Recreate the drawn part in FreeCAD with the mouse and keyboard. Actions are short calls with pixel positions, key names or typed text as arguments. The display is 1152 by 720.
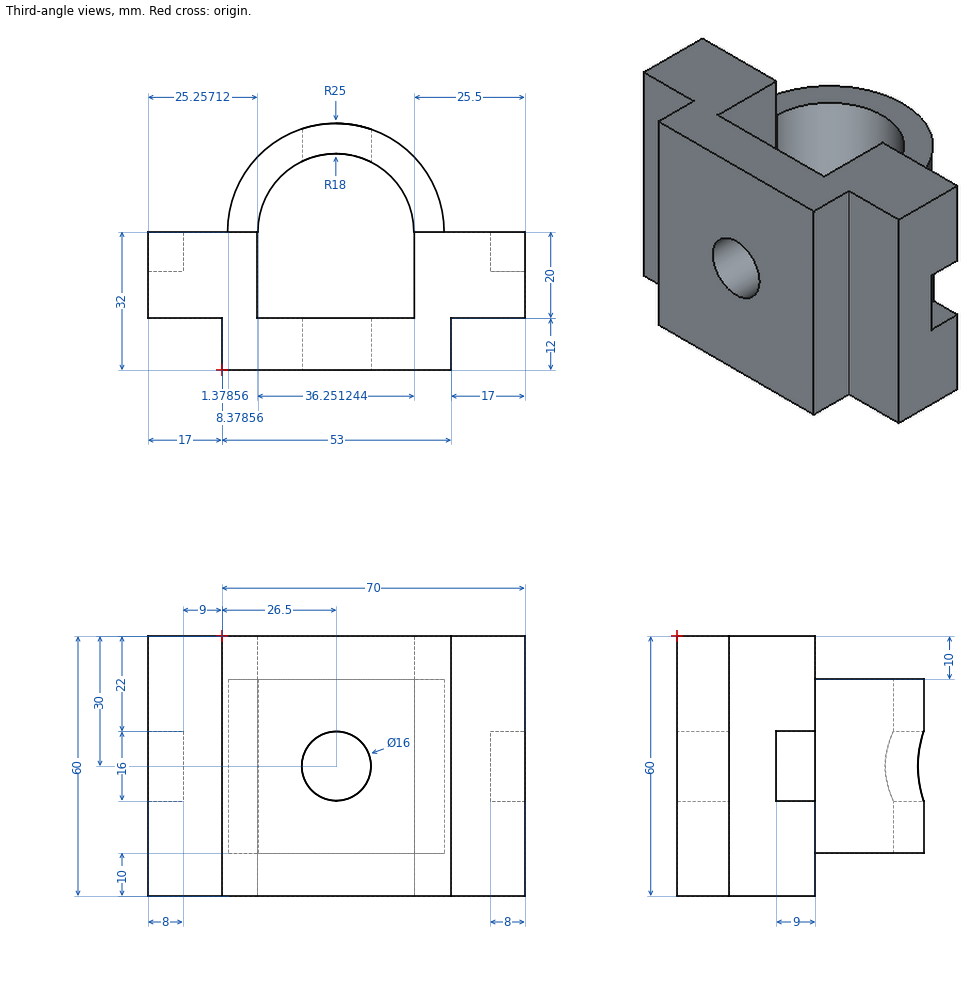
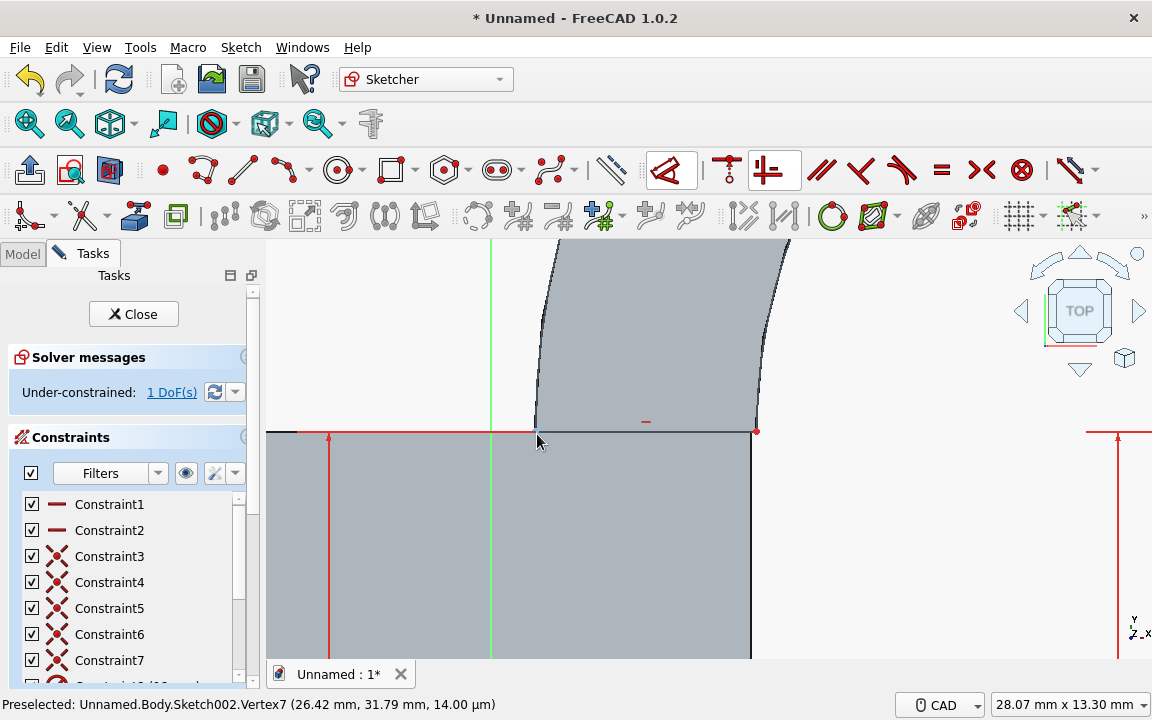
click(536, 432)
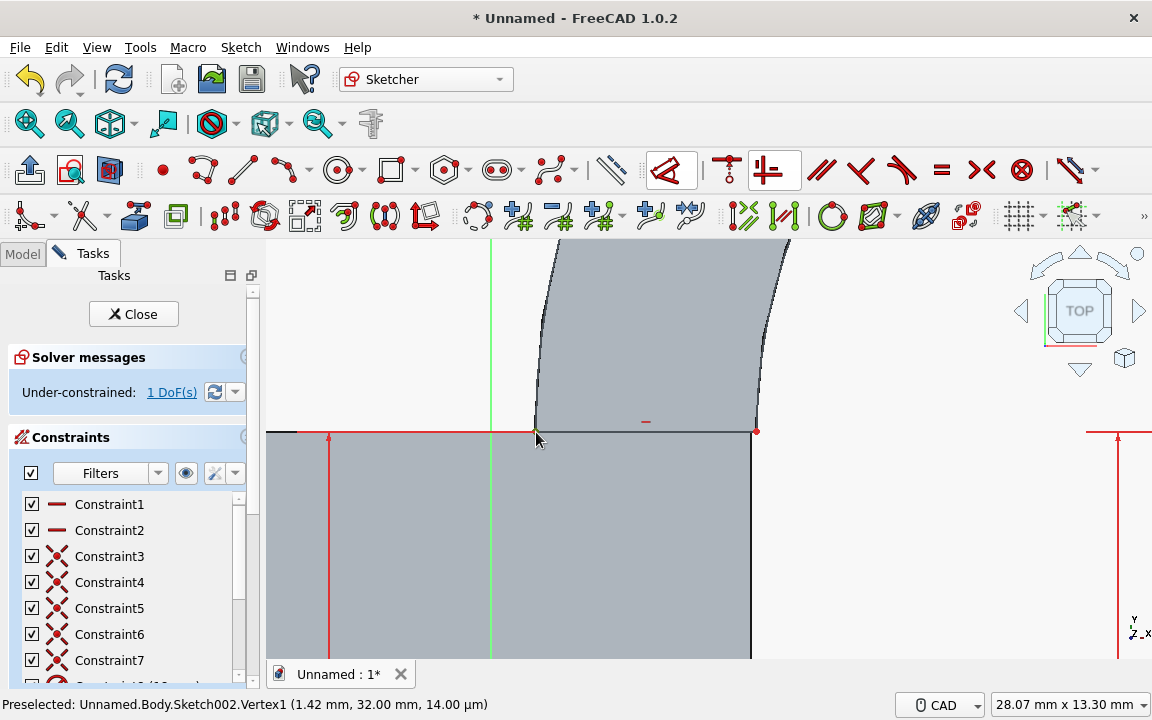
key(l)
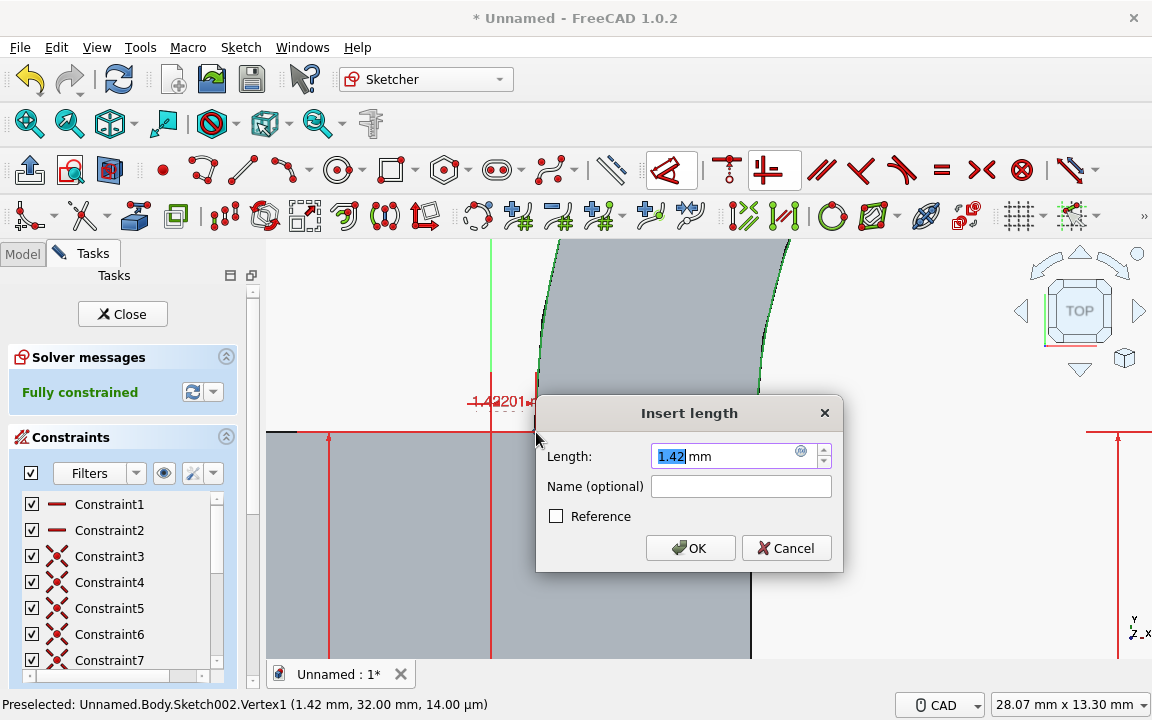
text(1.37856)
key(Return)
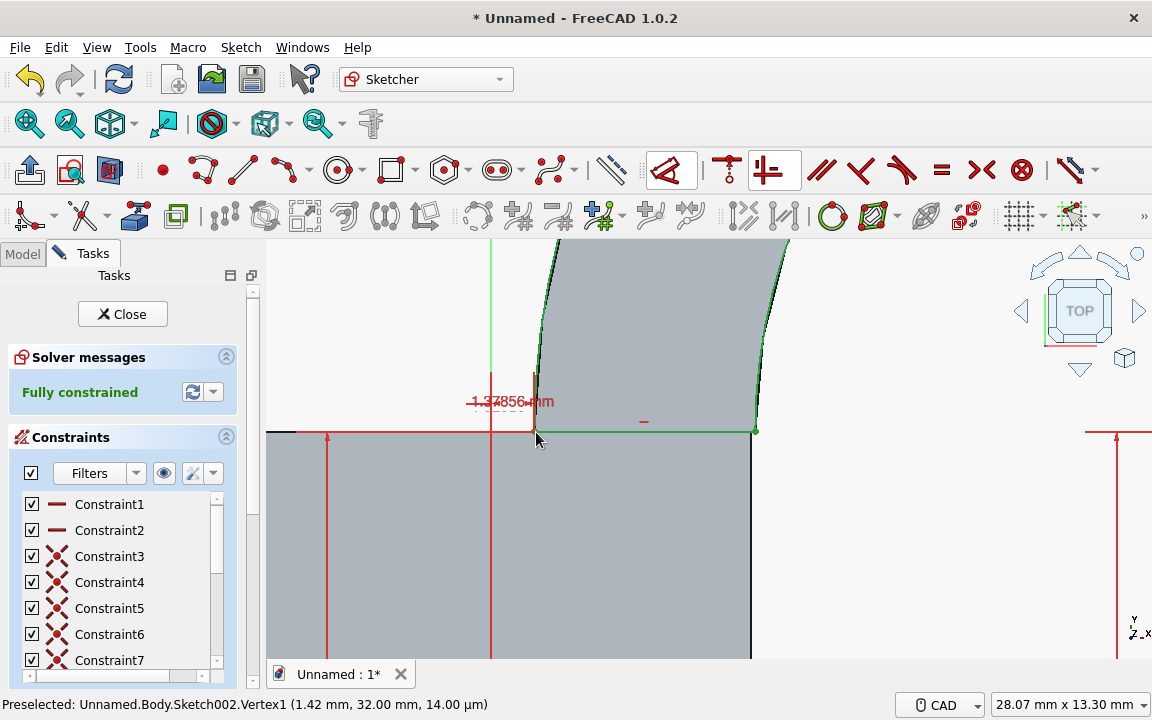
click(123, 314)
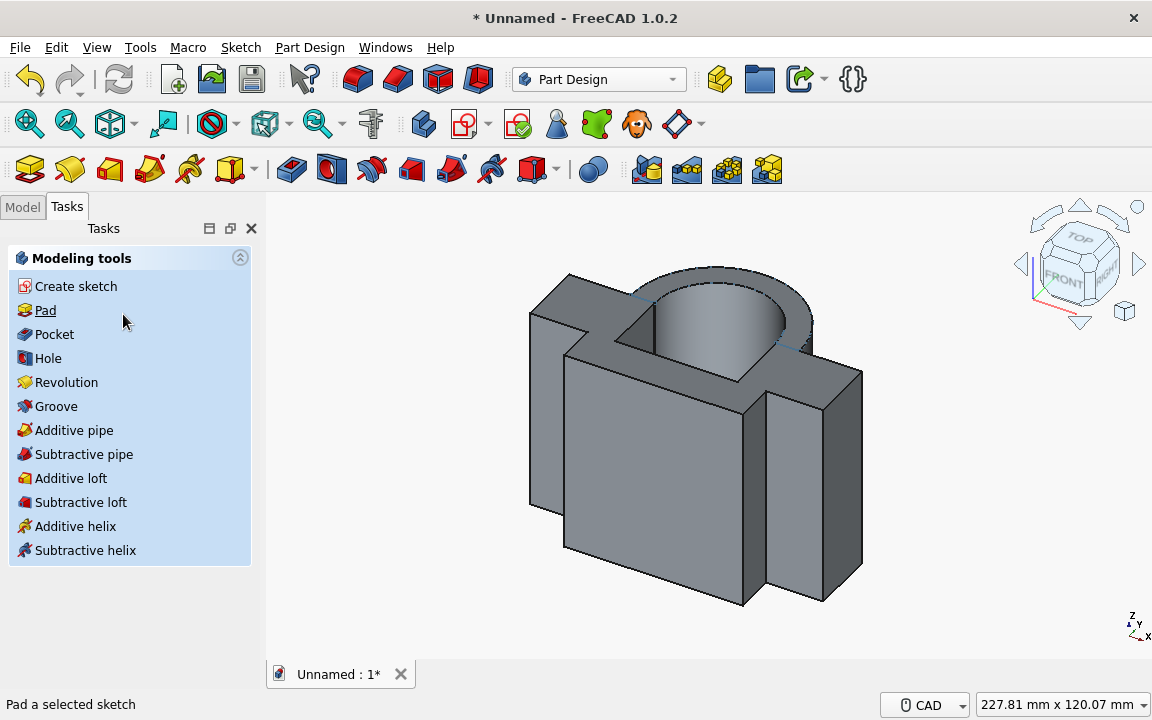
click(292, 170)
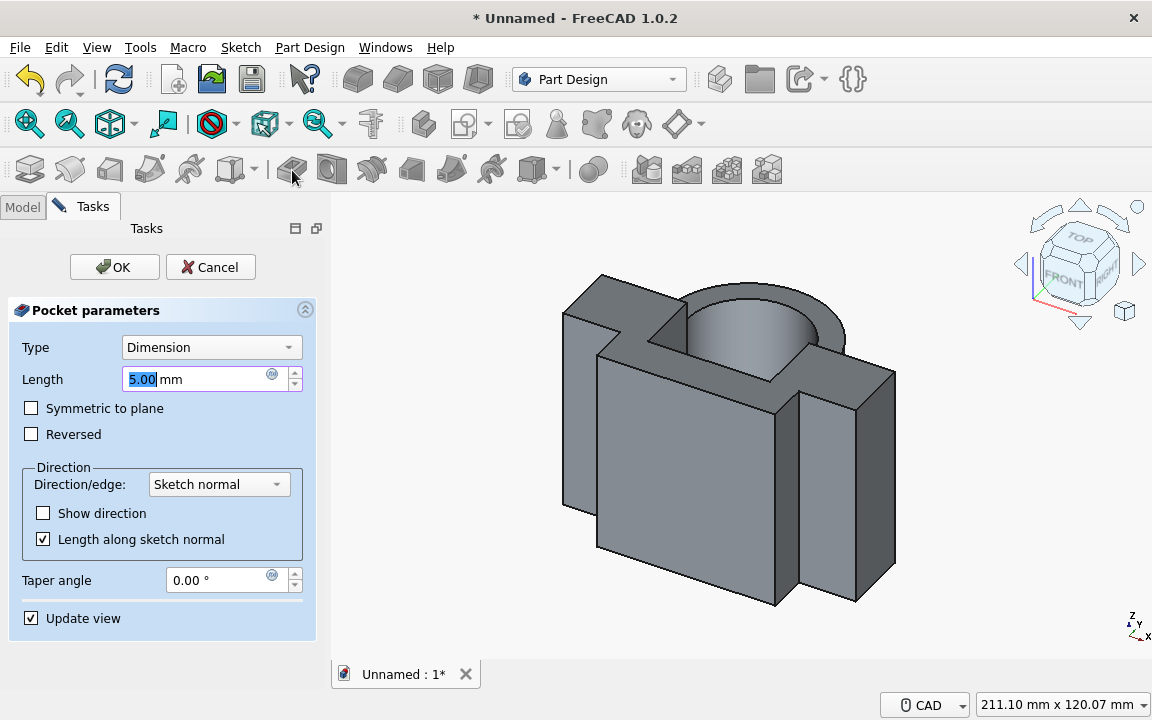
text(10)
key(Tab)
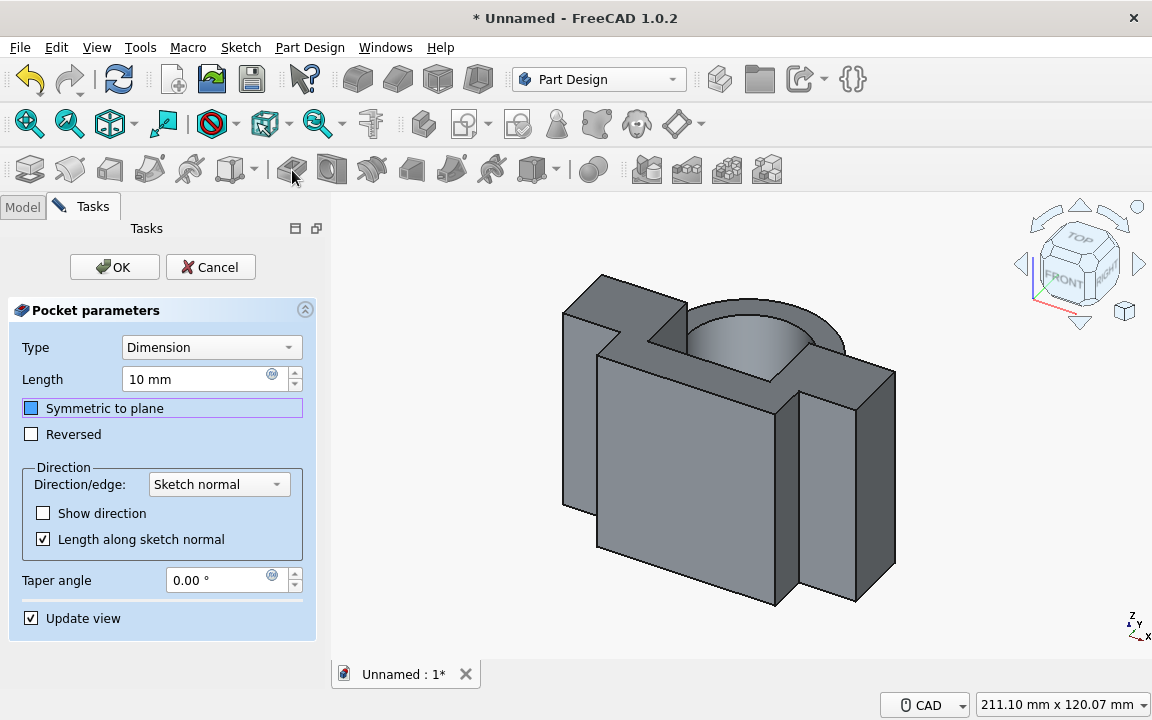
click(115, 267)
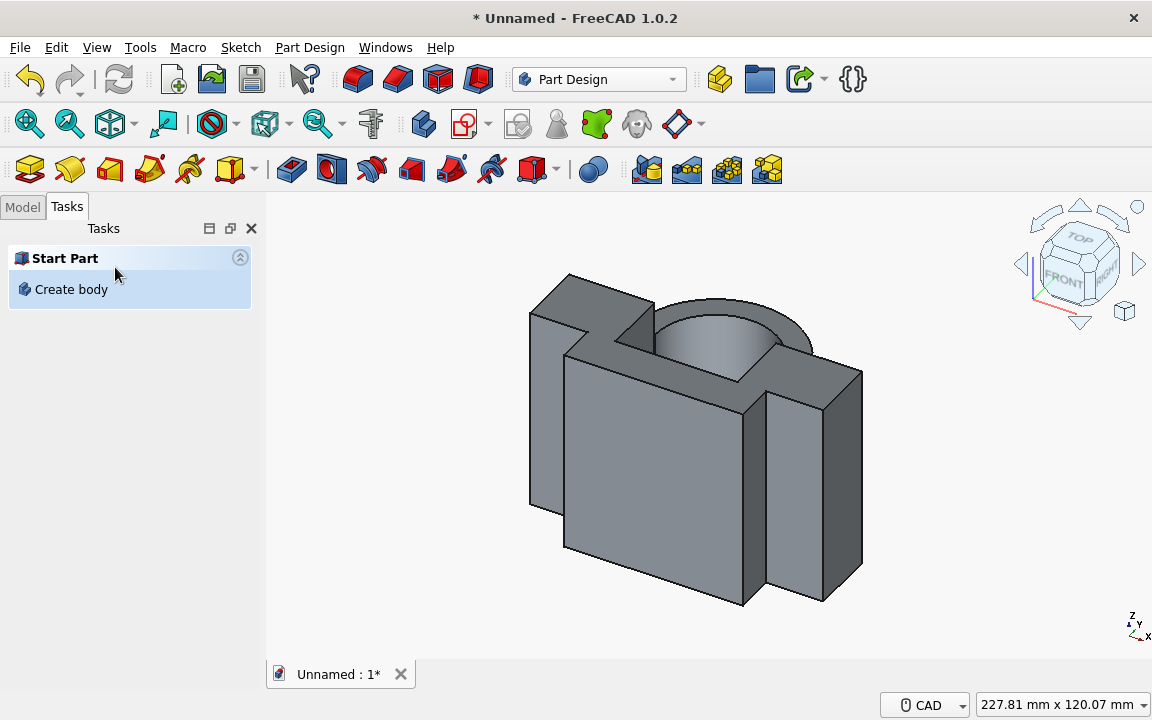
click(23, 206)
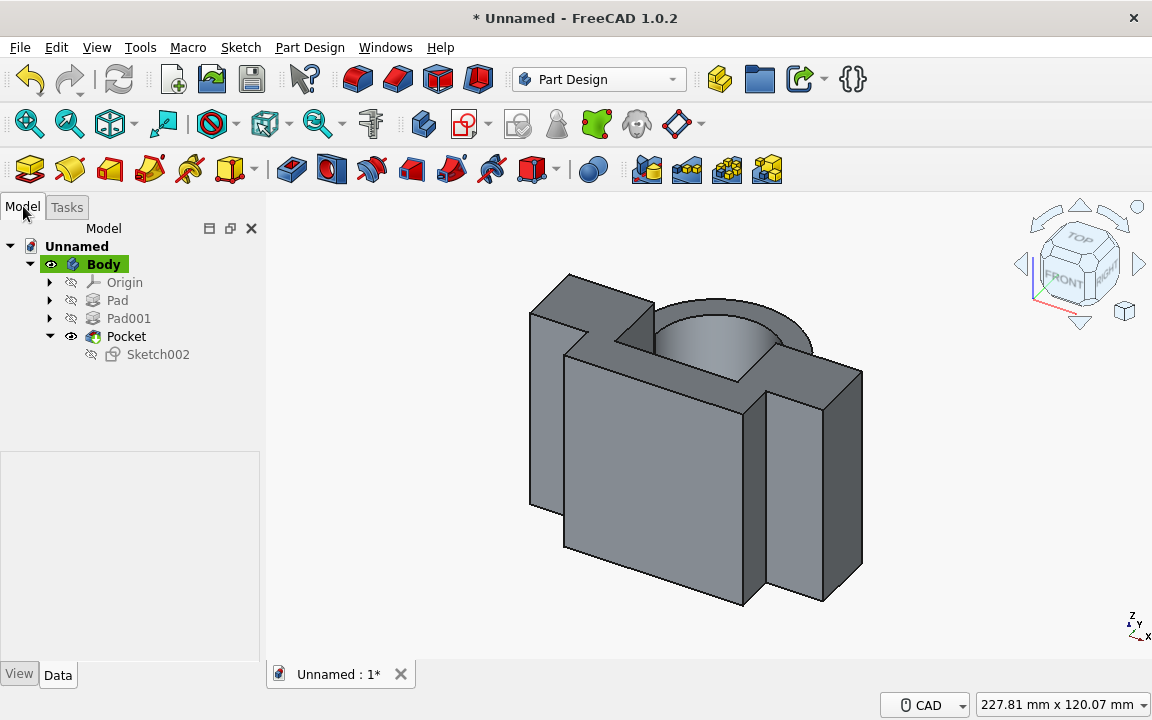
click(50, 282)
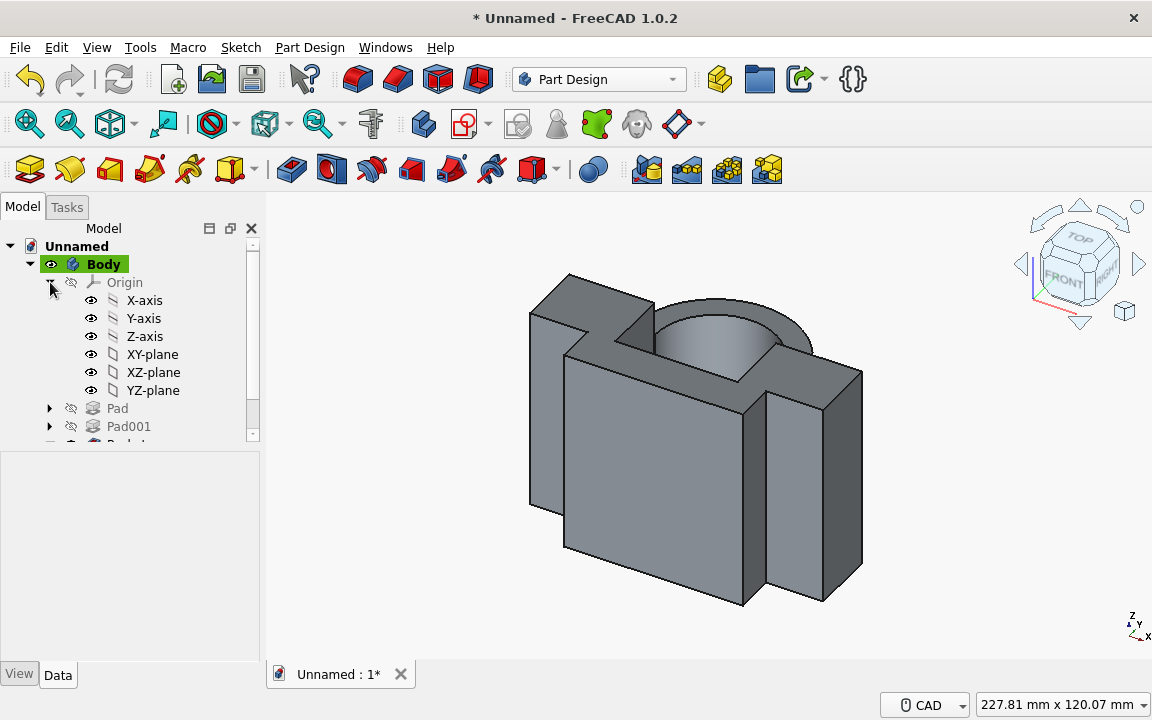
click(136, 354)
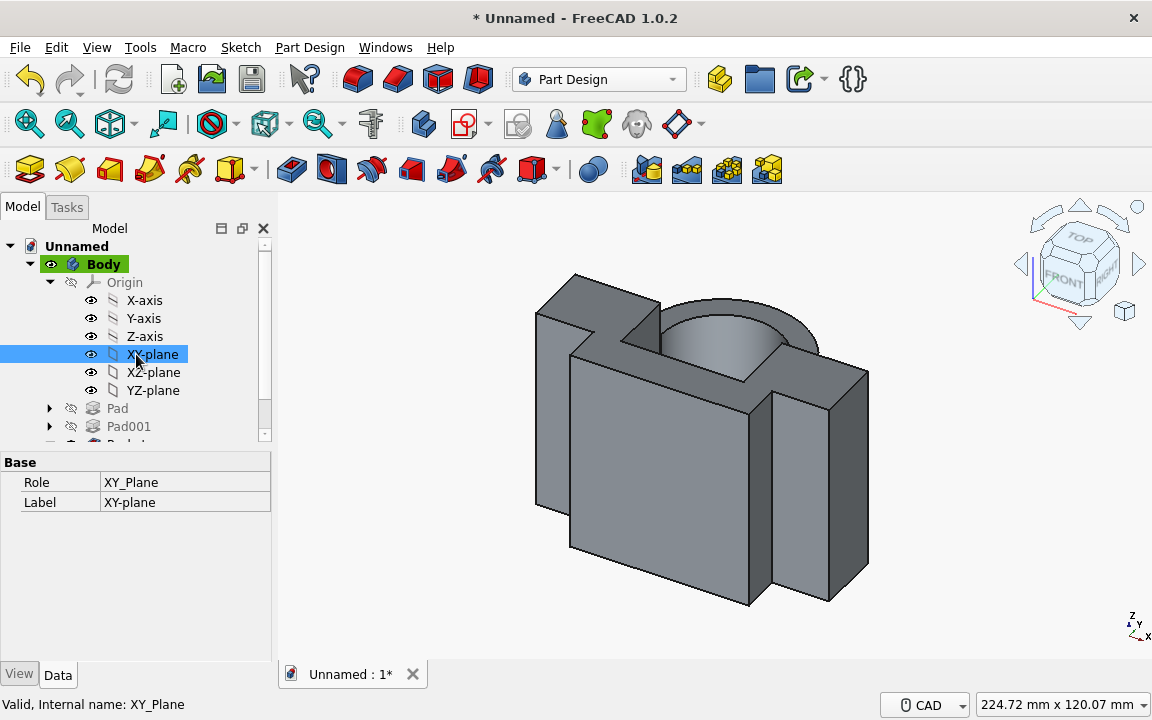
click(678, 124)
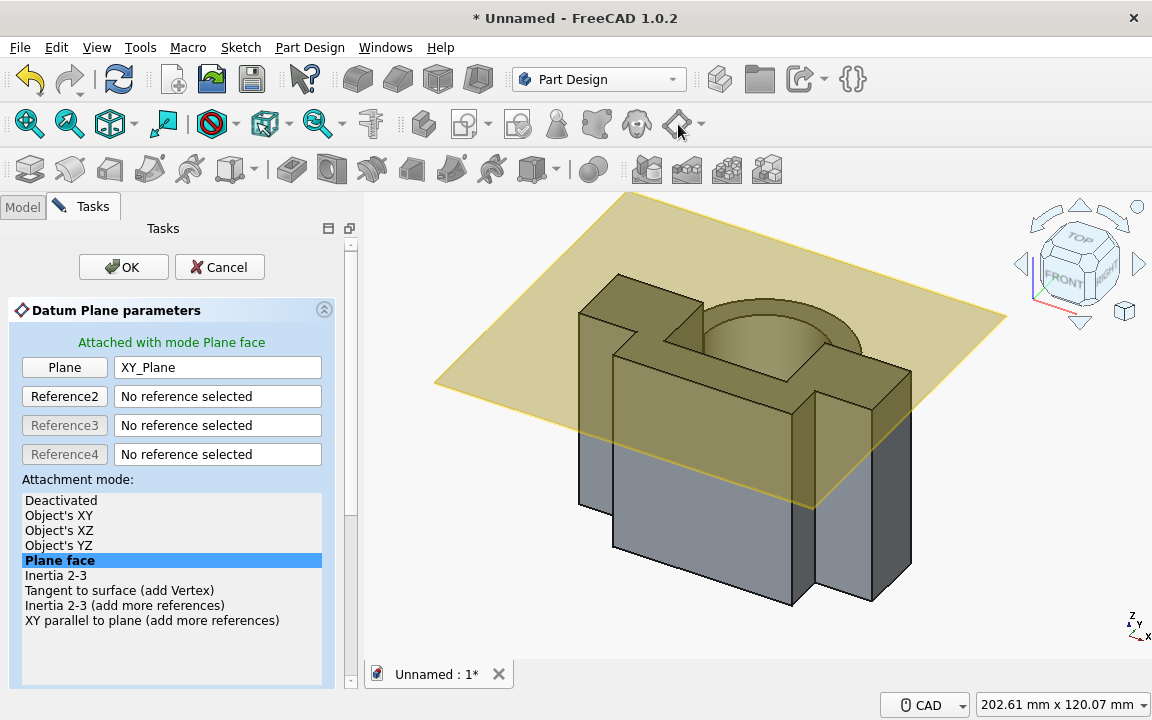
scroll(351, 463, down, 3)